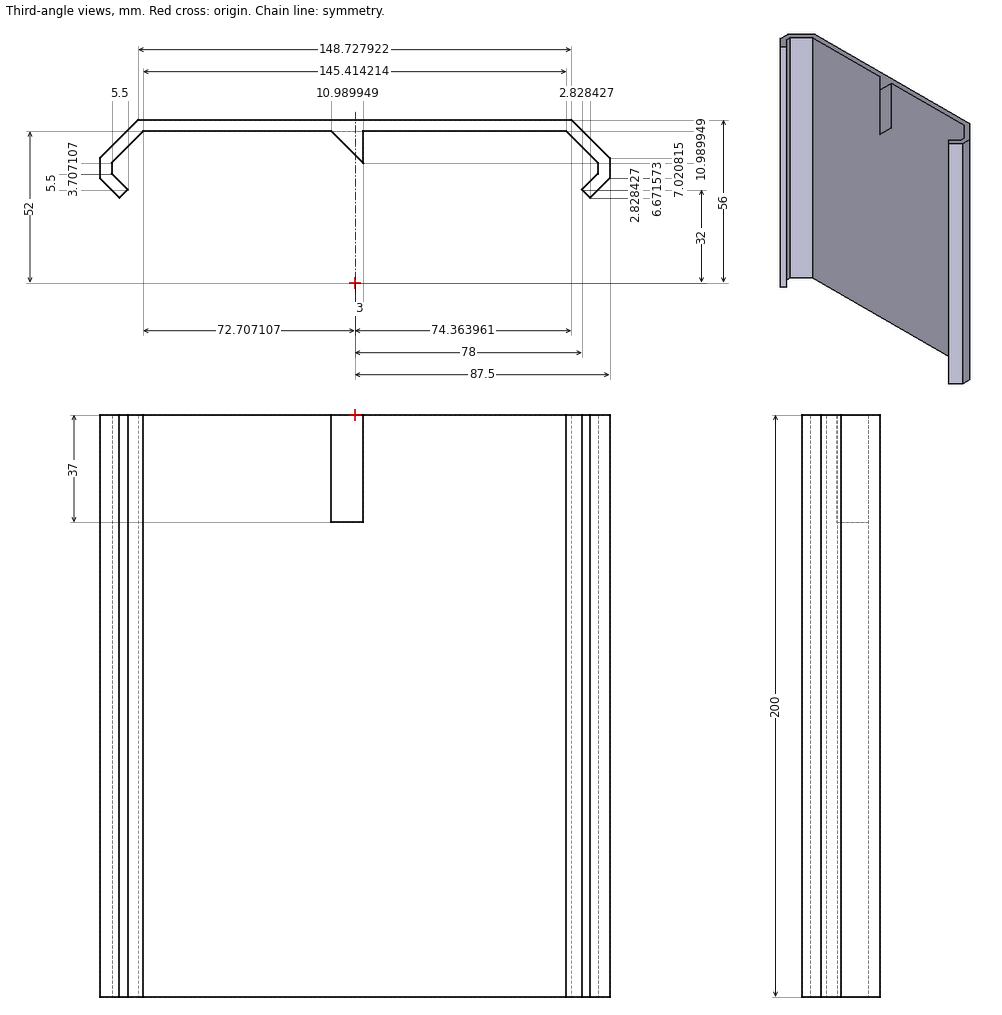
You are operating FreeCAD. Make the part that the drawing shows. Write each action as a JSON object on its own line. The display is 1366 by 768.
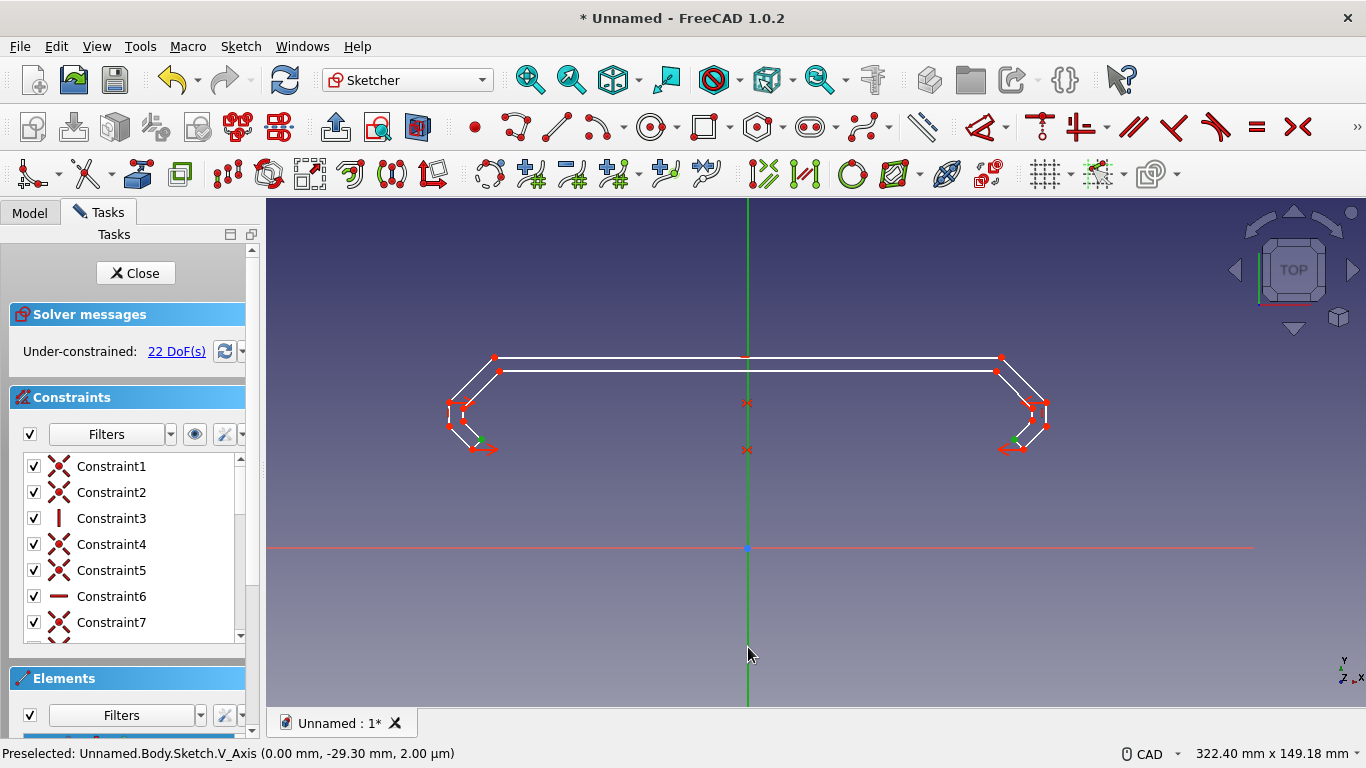
{"action": "left_click", "coordinate": [1298, 128]}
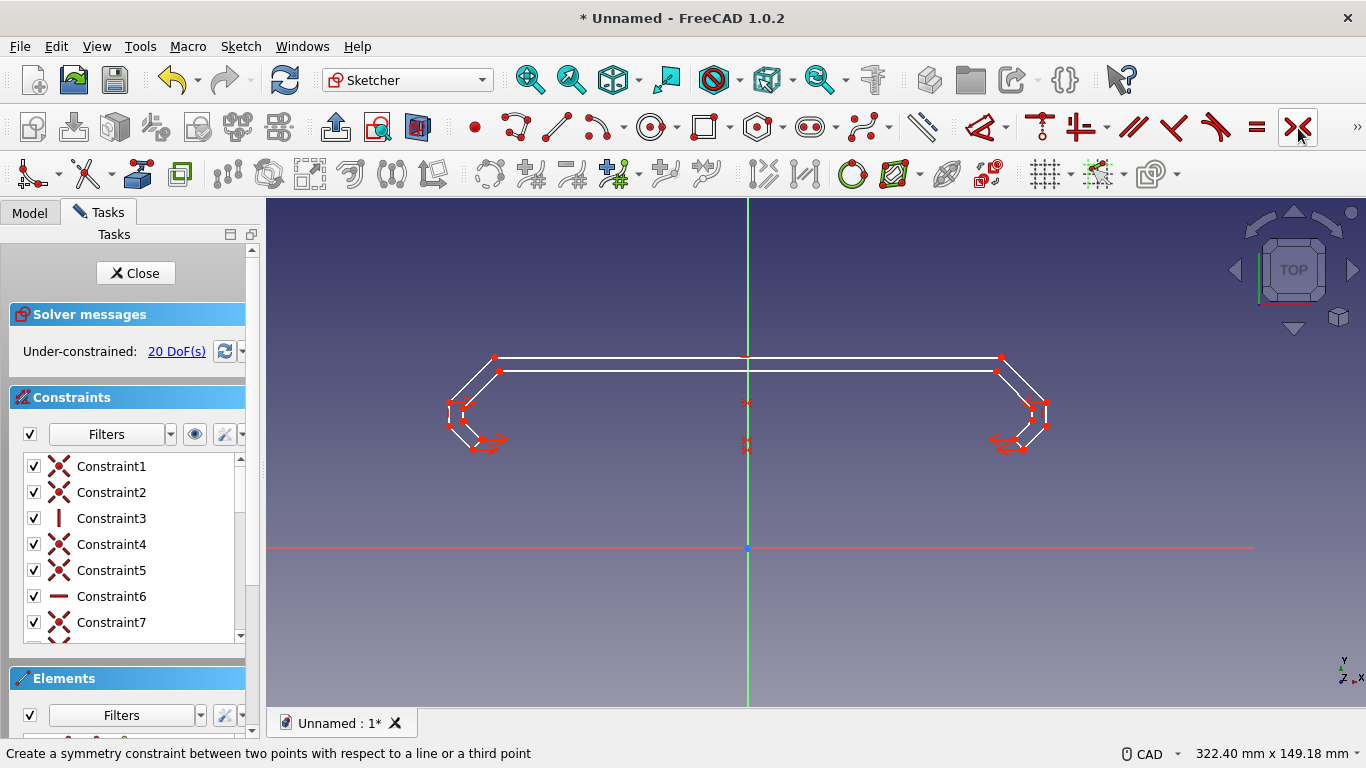
{"action": "left_click", "coordinate": [463, 408]}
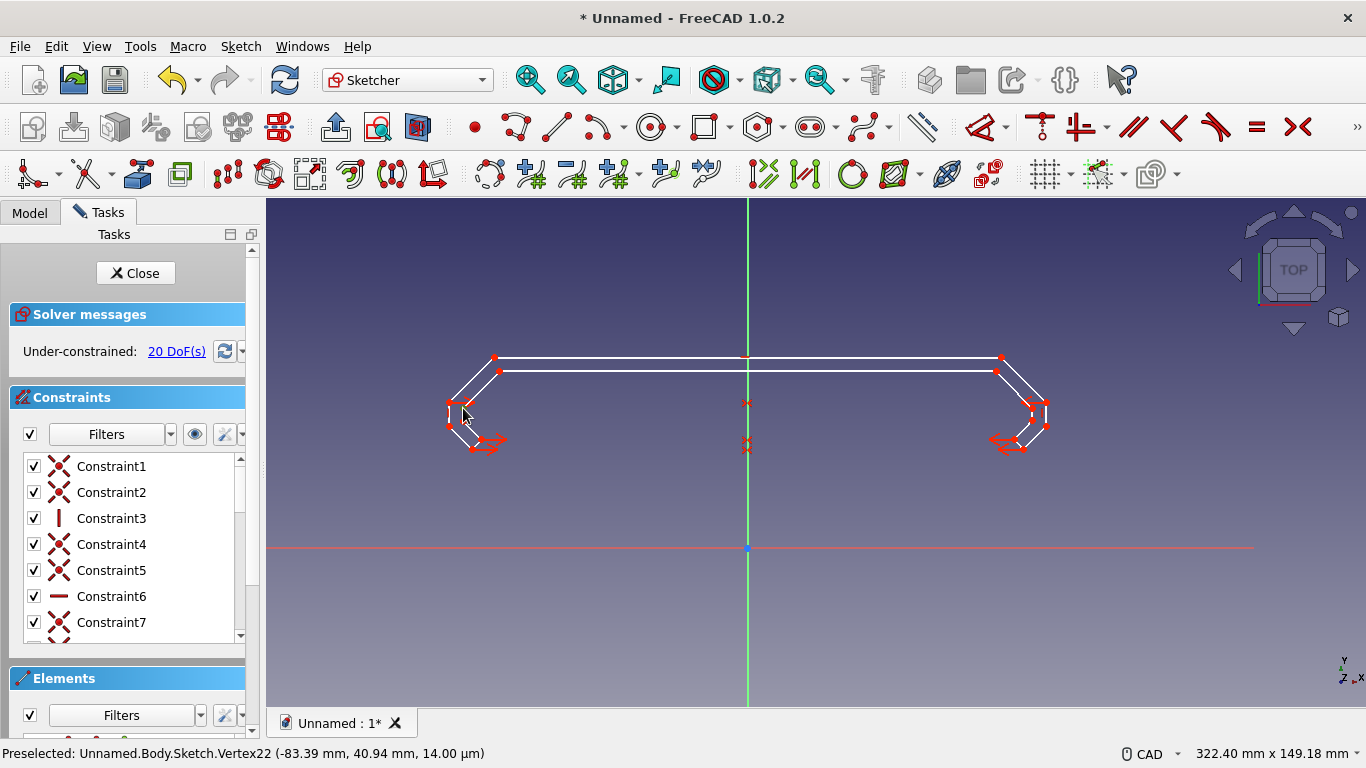
{"action": "left_click", "coordinate": [1032, 409]}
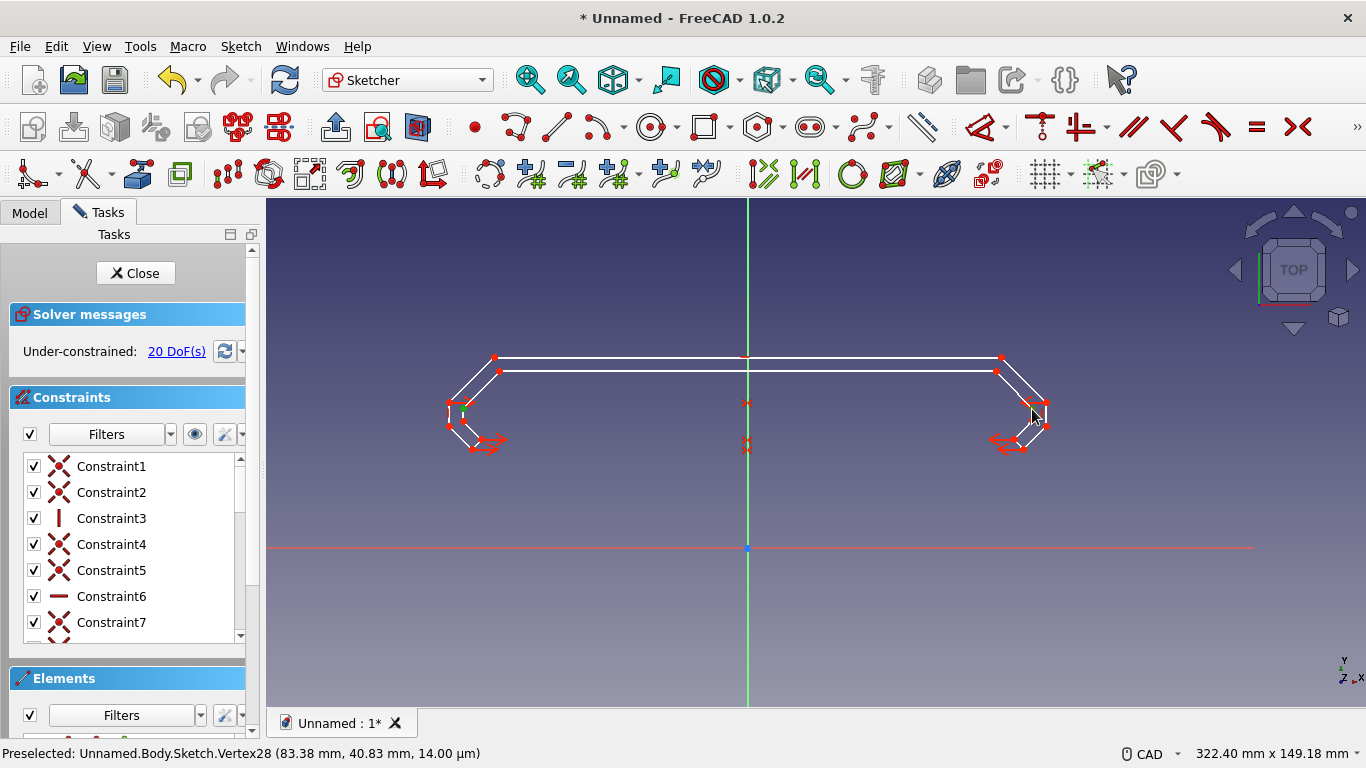
{"action": "left_click", "coordinate": [748, 647]}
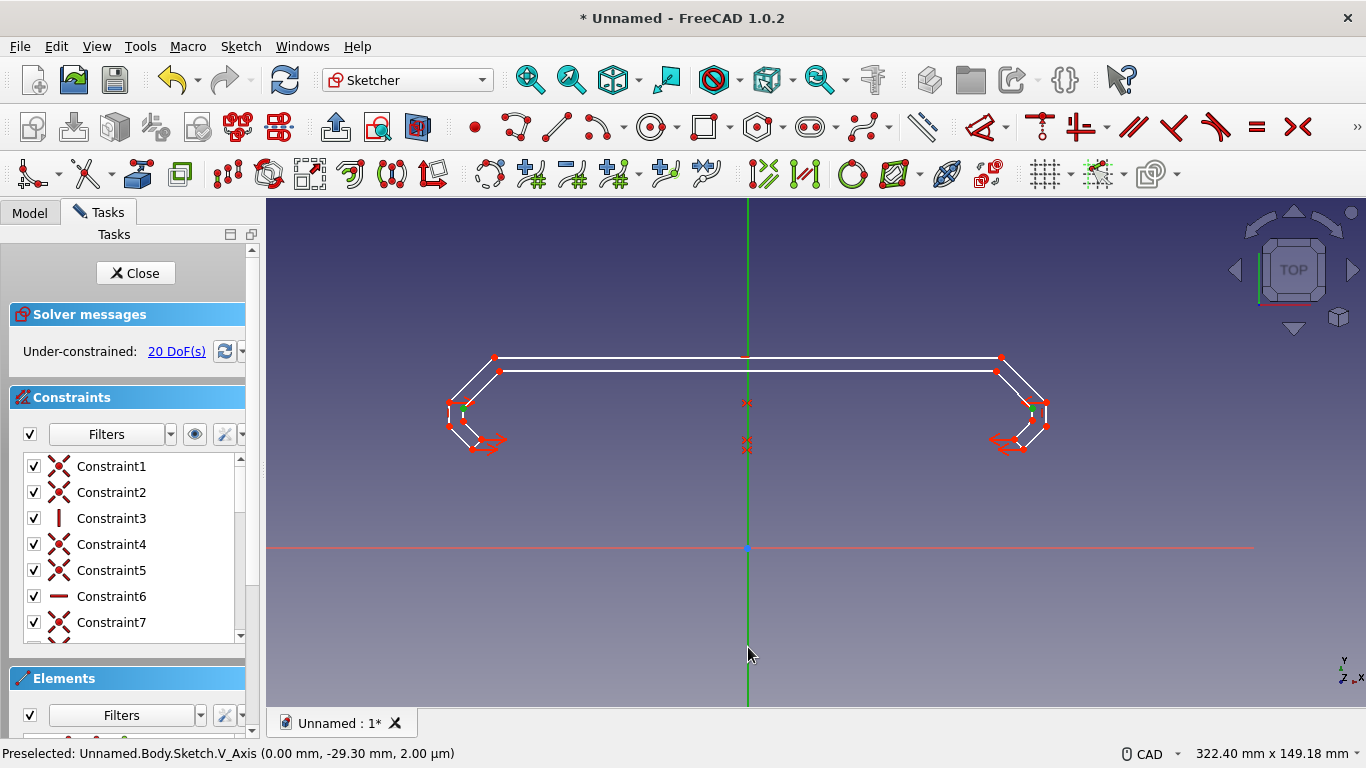
{"action": "left_click", "coordinate": [1298, 128]}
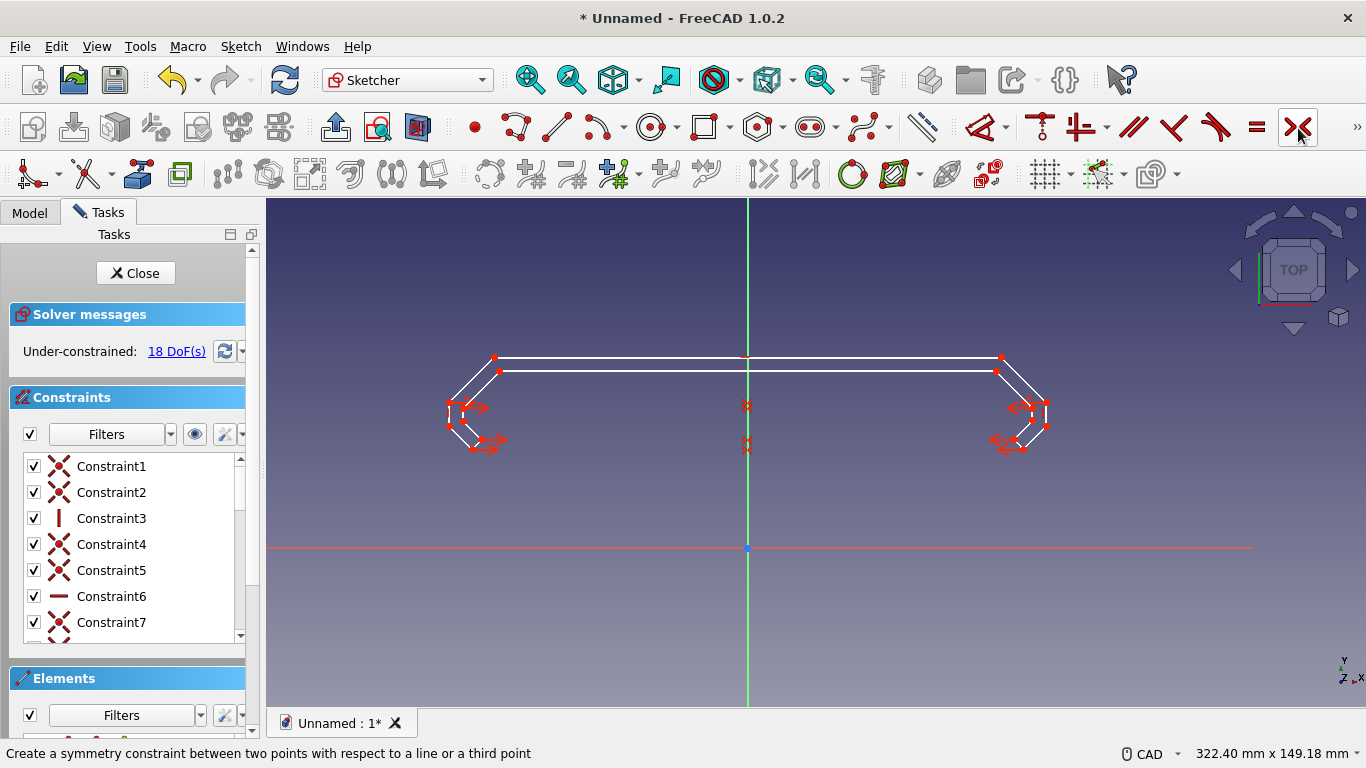
{"action": "left_click", "coordinate": [1014, 440]}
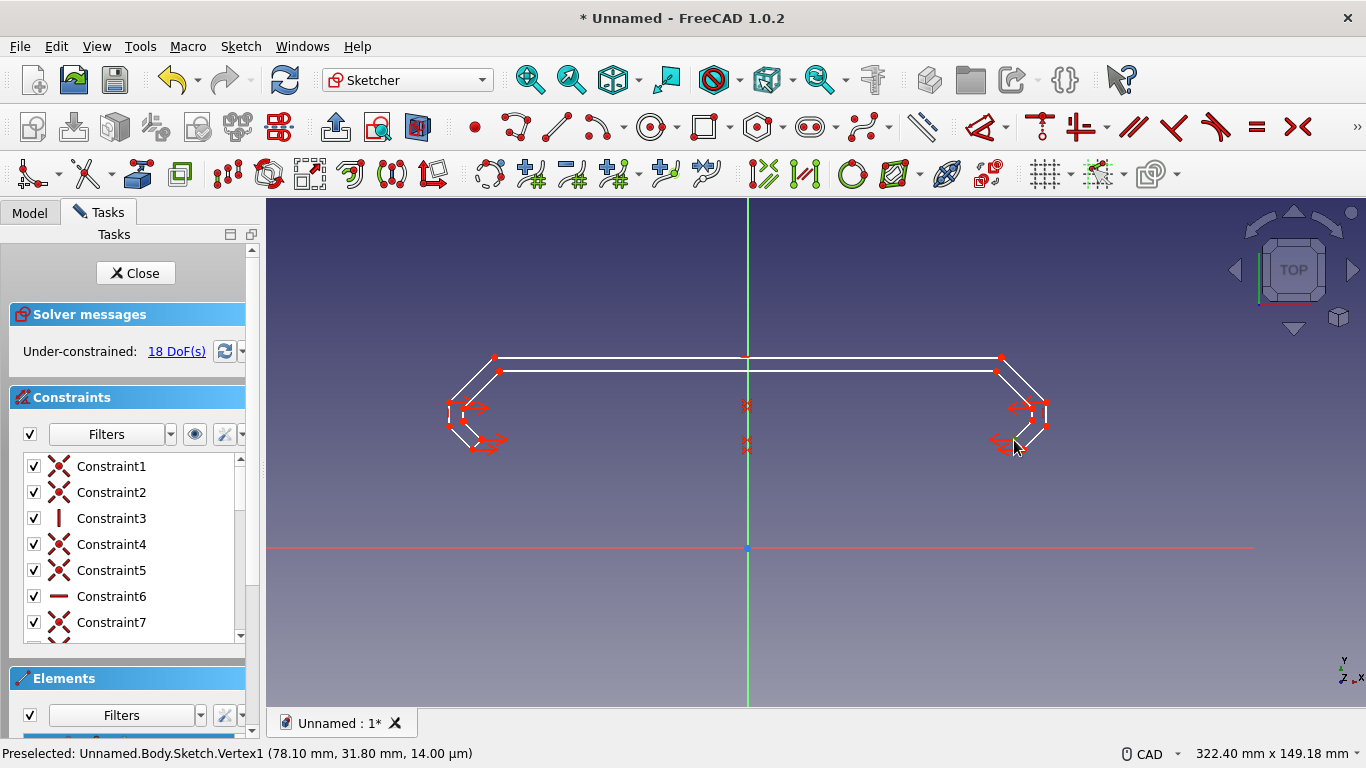
{"action": "left_click", "coordinate": [1006, 128]}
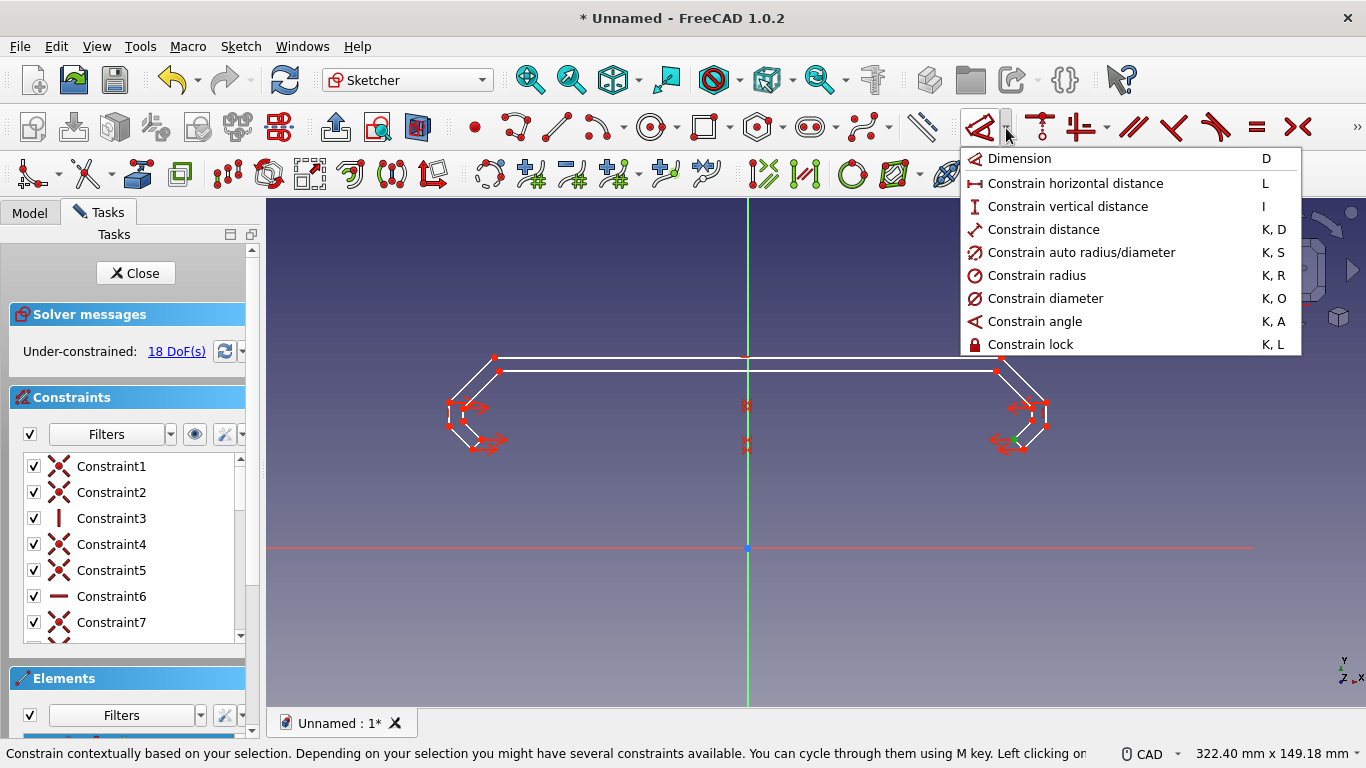
{"action": "left_click", "coordinate": [1131, 184]}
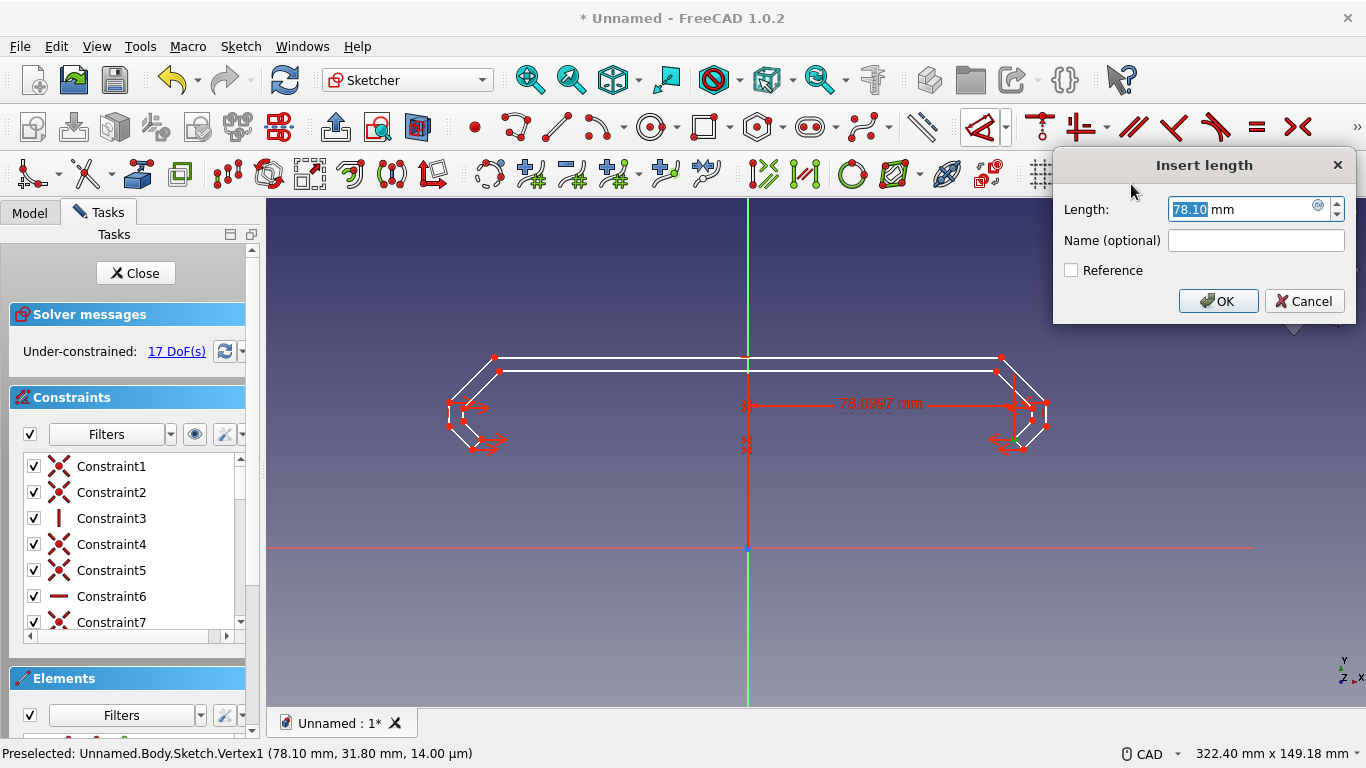
{"action": "type", "text": "78"}
{"action": "key", "text": "Return"}